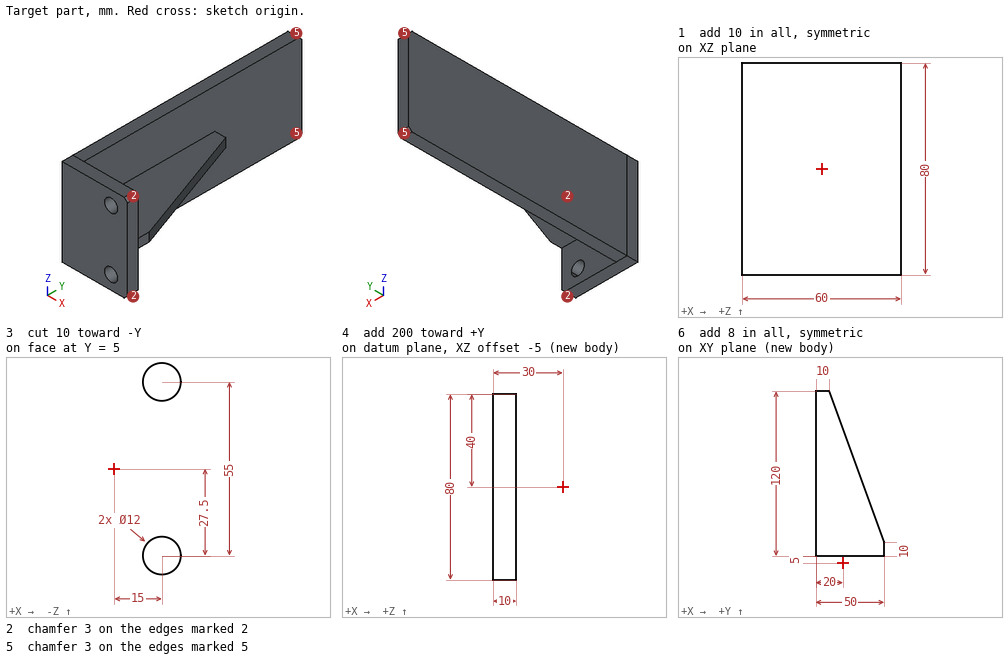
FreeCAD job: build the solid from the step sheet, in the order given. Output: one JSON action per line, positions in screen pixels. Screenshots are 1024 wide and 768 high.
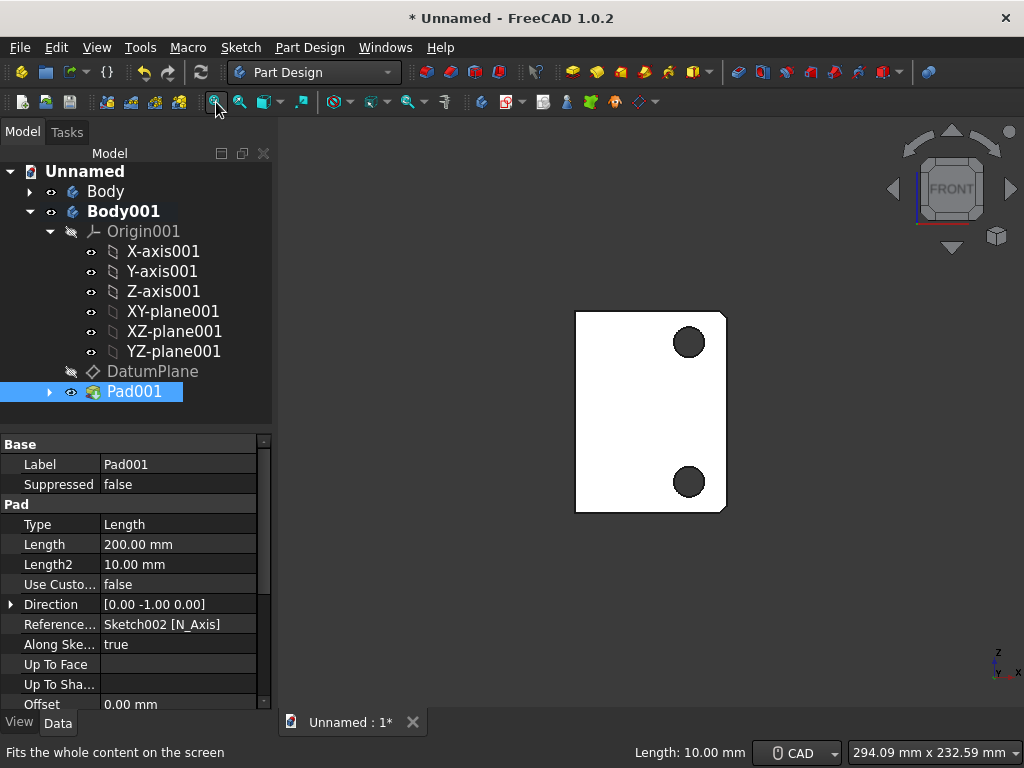
{"action": "key", "text": "3"}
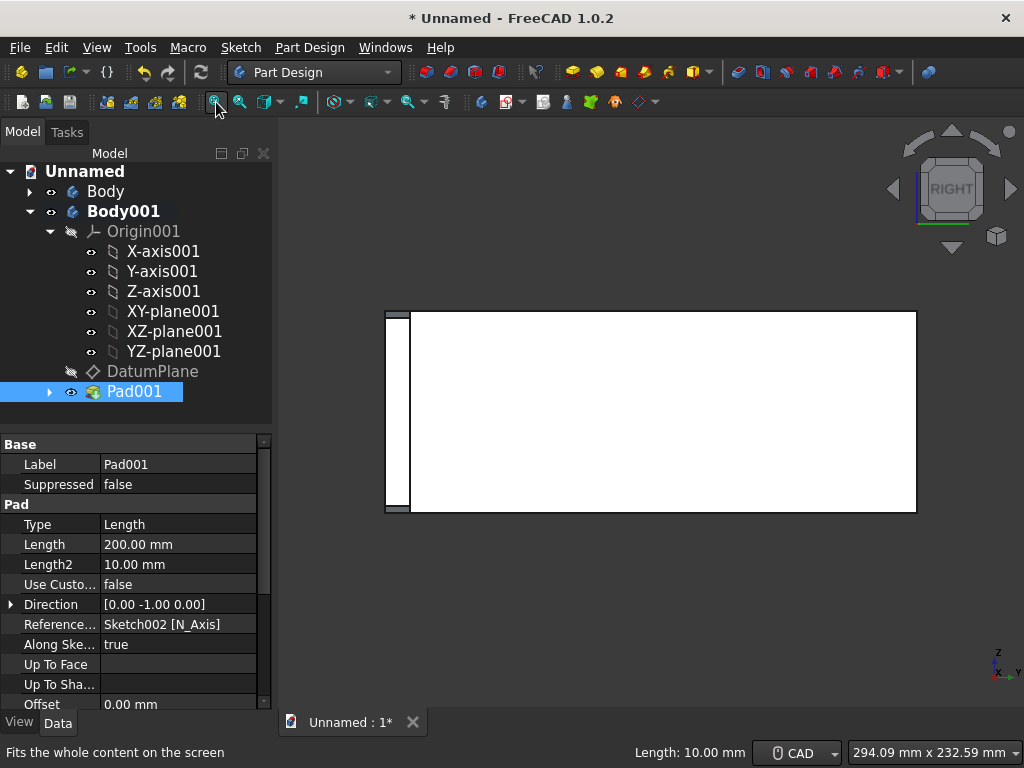
{"action": "key", "text": "5"}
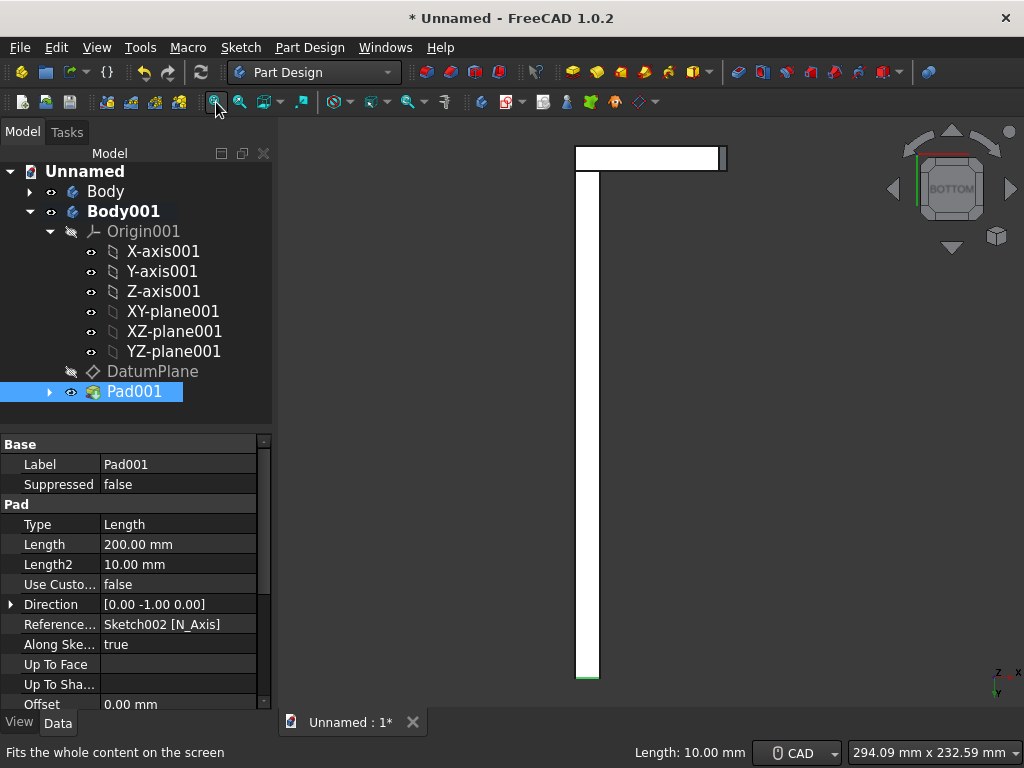
{"action": "key", "text": "4"}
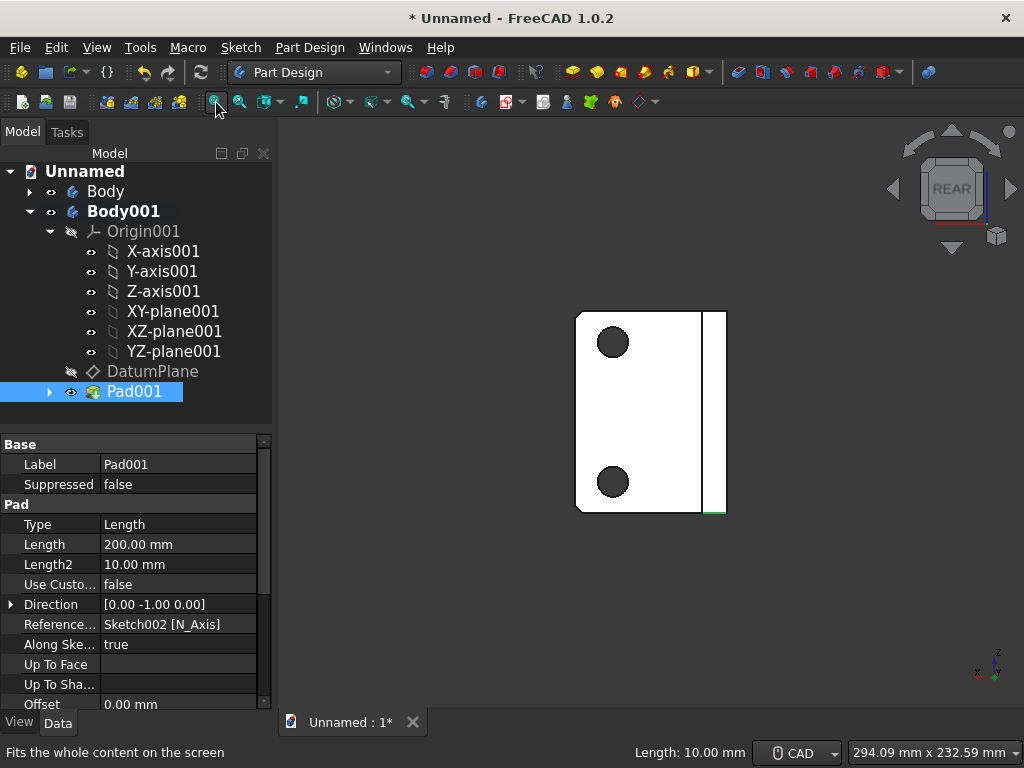
{"action": "left_click", "coordinate": [216, 102]}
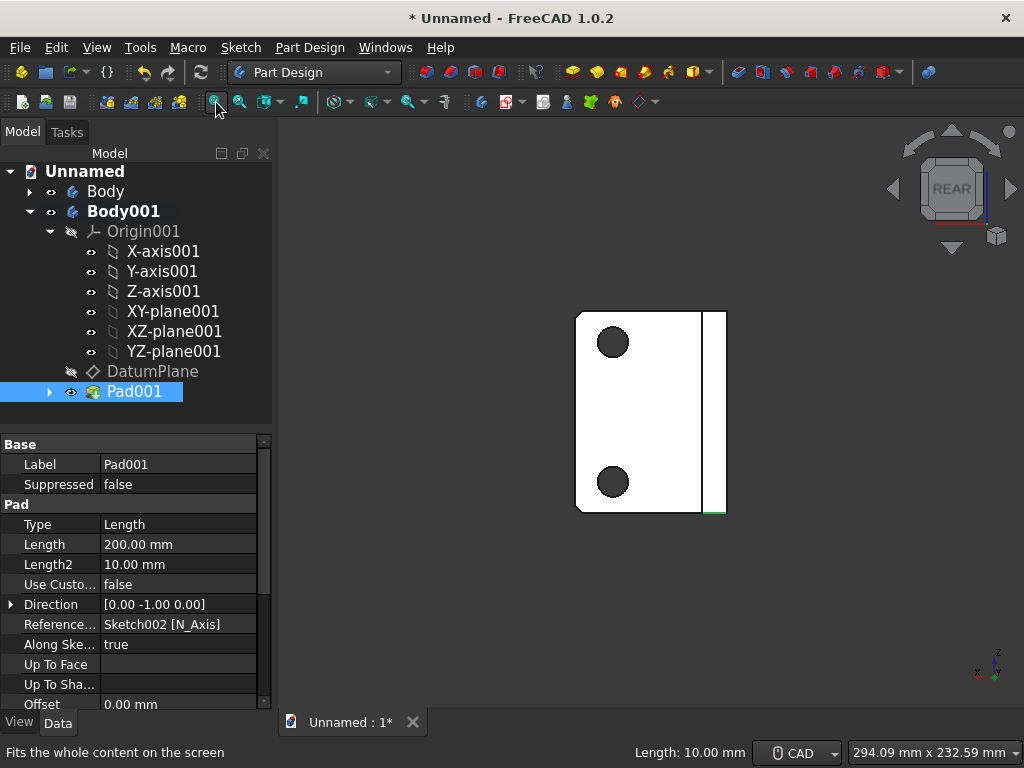
{"action": "key", "text": "6"}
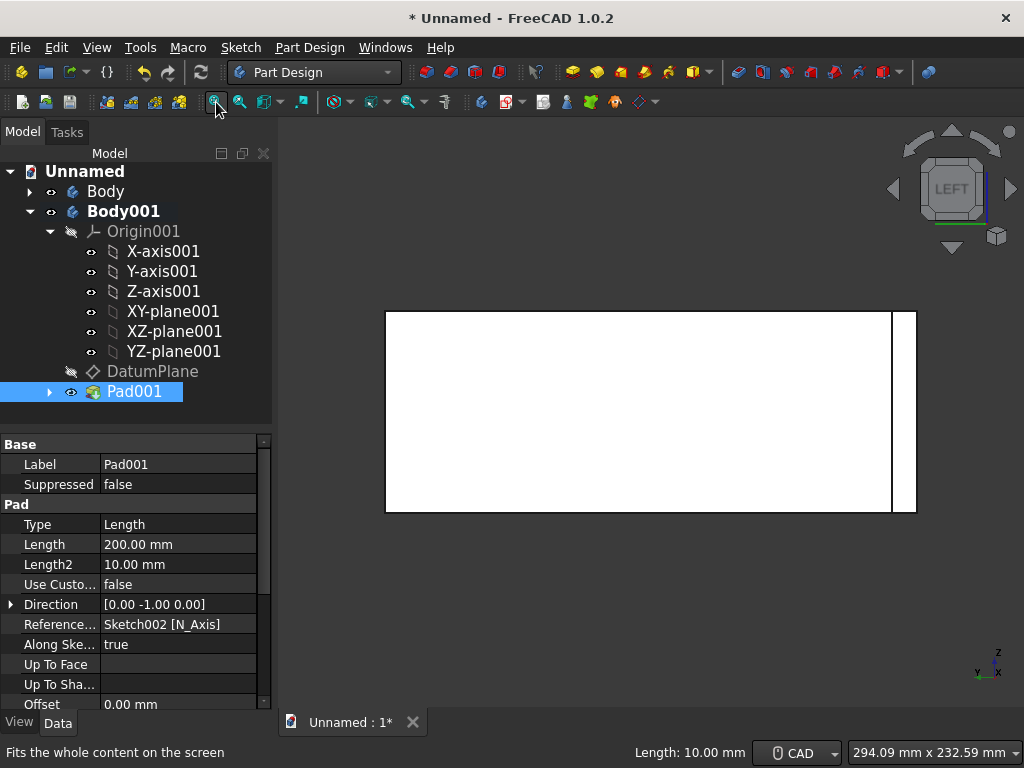
{"action": "key", "text": "v 3"}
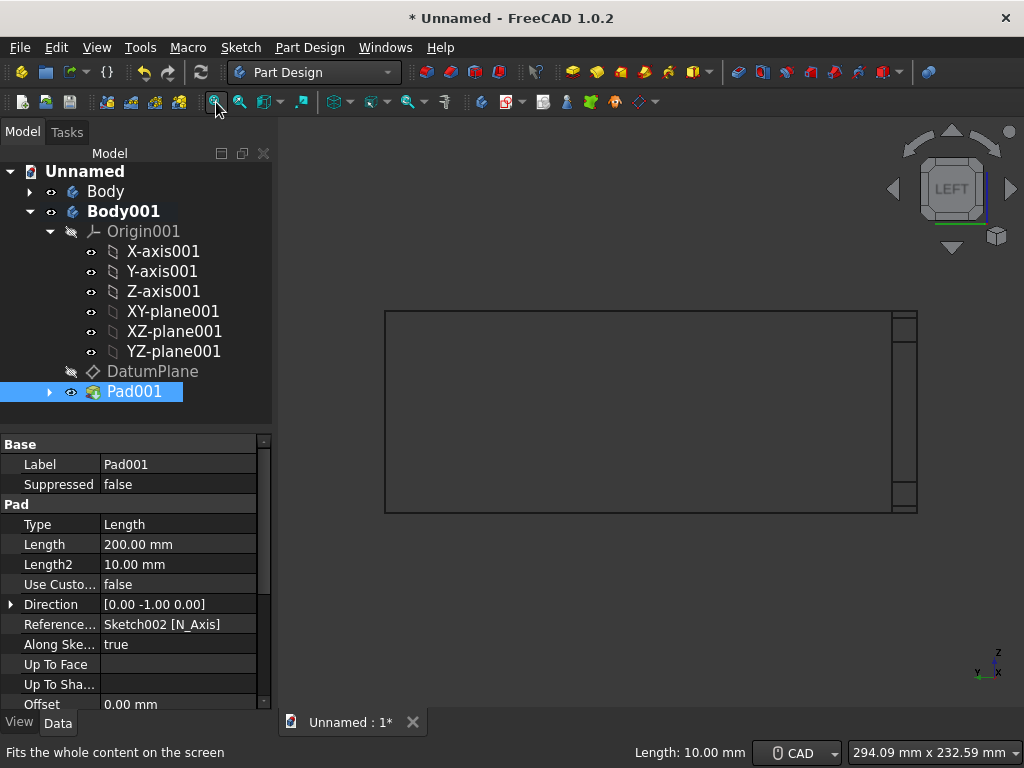
{"action": "key", "text": "0"}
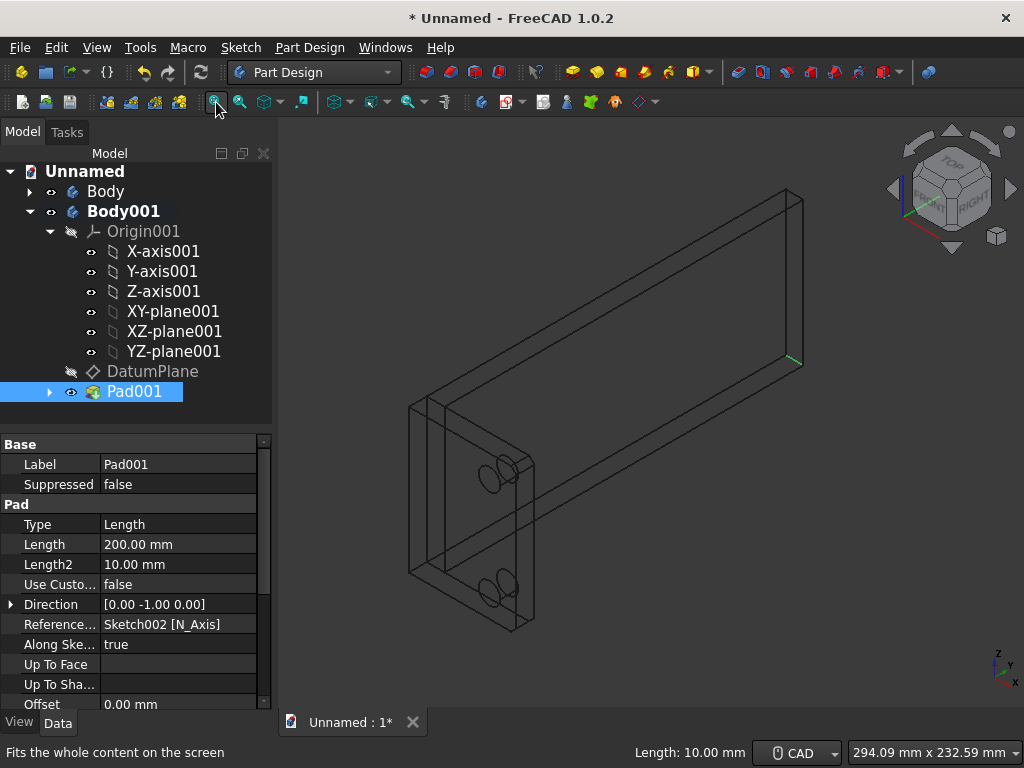
{"action": "left_click", "coordinate": [794, 194], "text": "ctrl"}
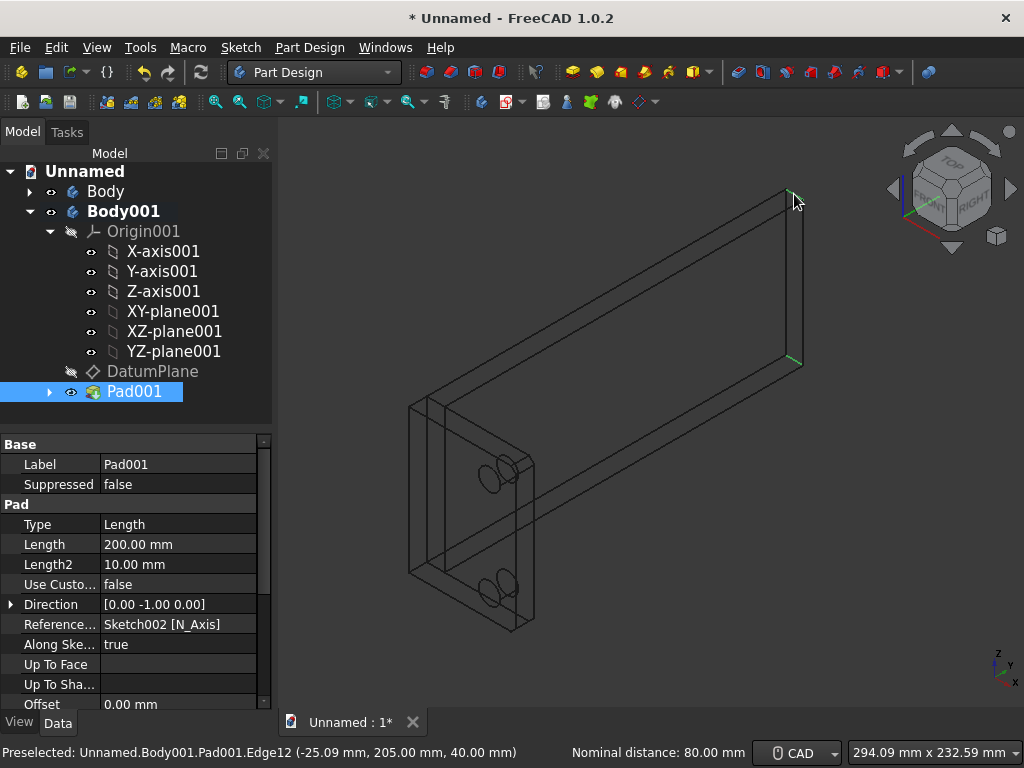
{"action": "key", "text": "v 1"}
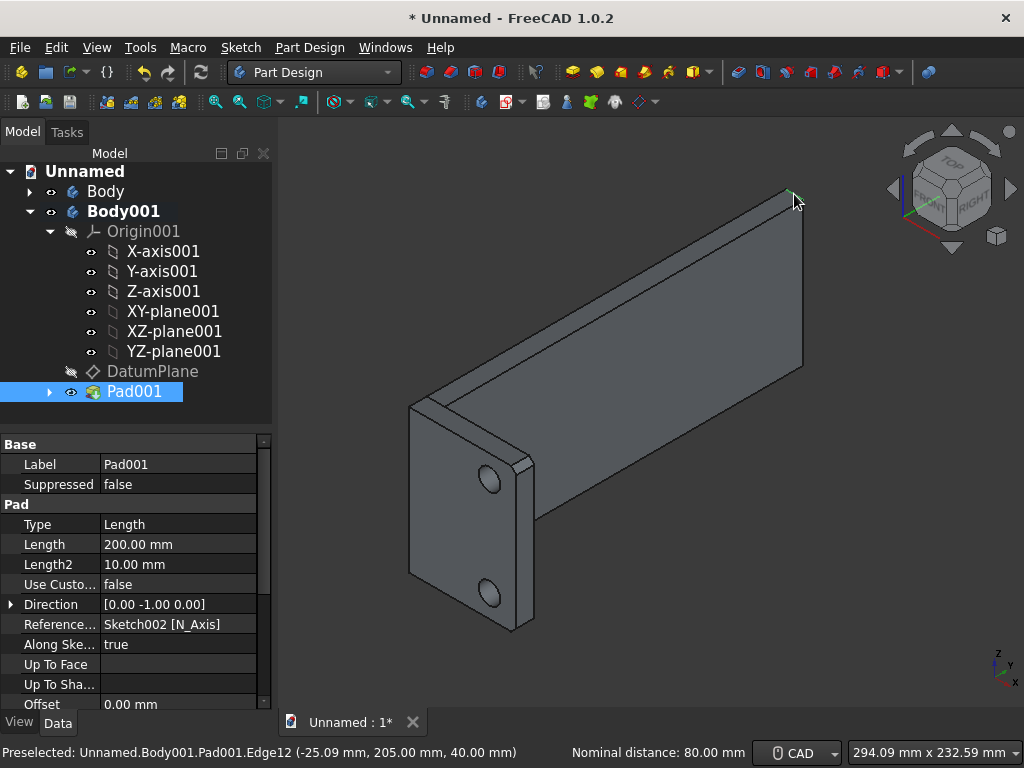
{"action": "left_click", "coordinate": [452, 72]}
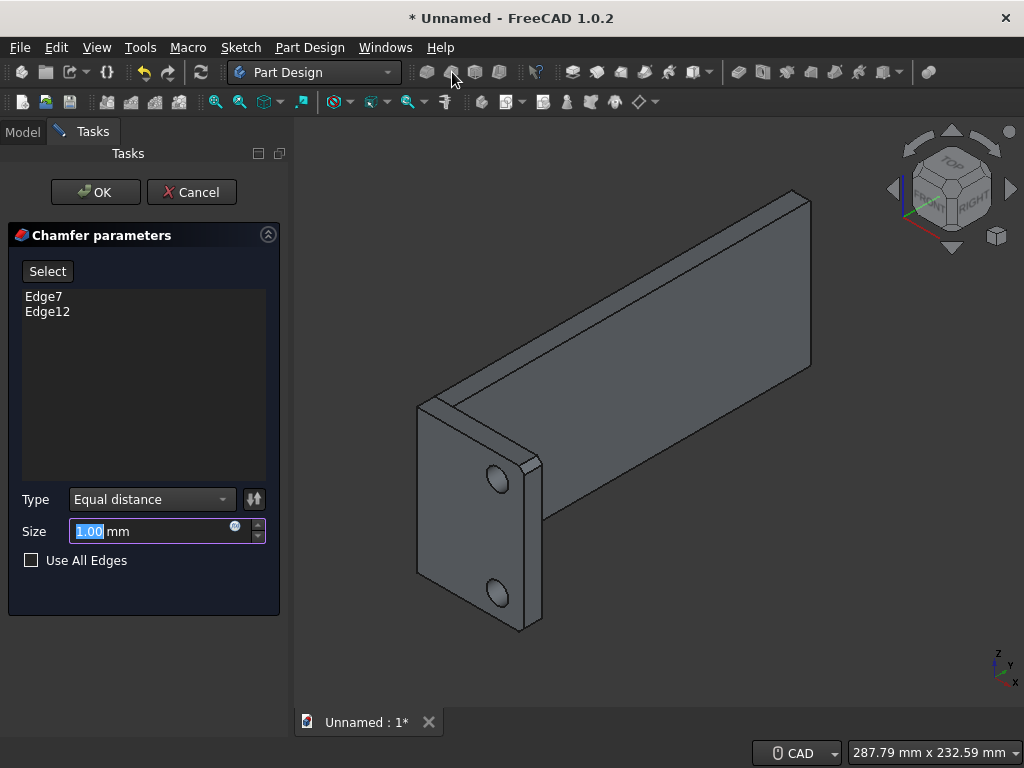
{"action": "type", "text": "3"}
{"action": "key", "text": "Tab"}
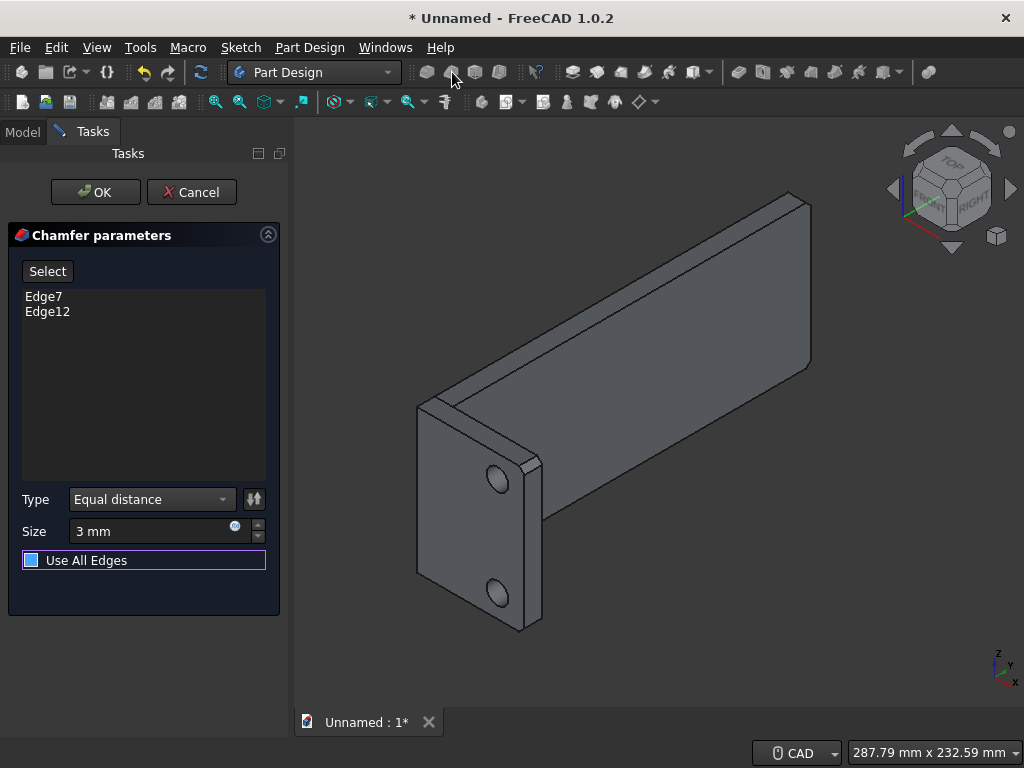
{"action": "left_click", "coordinate": [96, 192]}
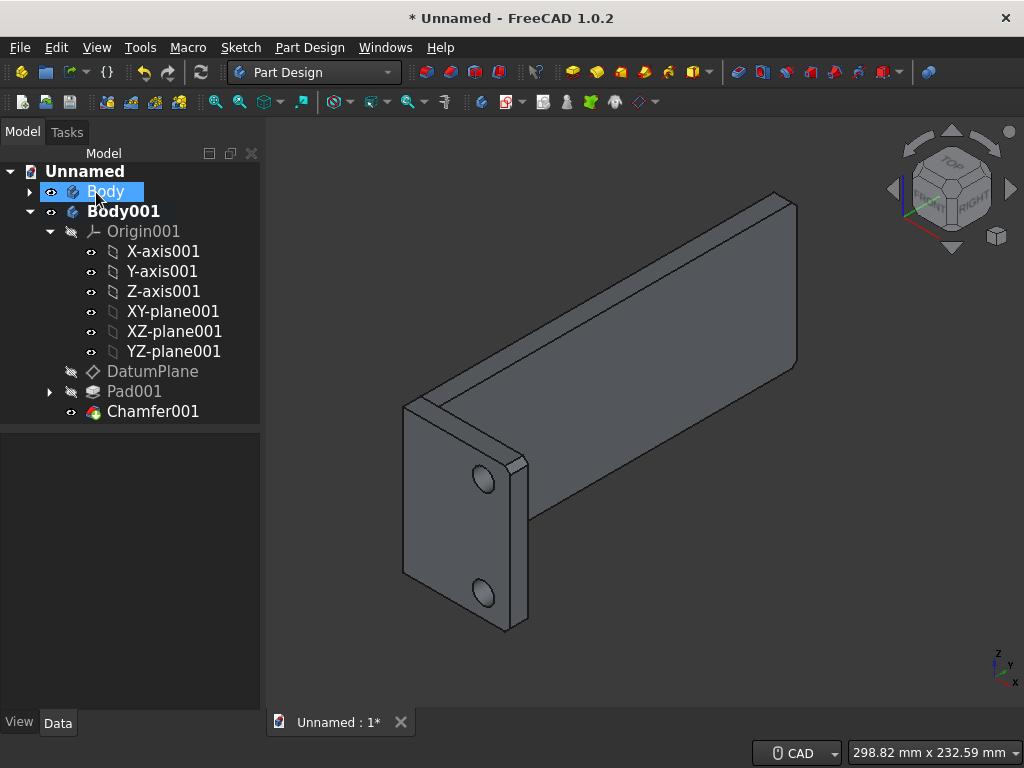
{"action": "left_click", "coordinate": [482, 102]}